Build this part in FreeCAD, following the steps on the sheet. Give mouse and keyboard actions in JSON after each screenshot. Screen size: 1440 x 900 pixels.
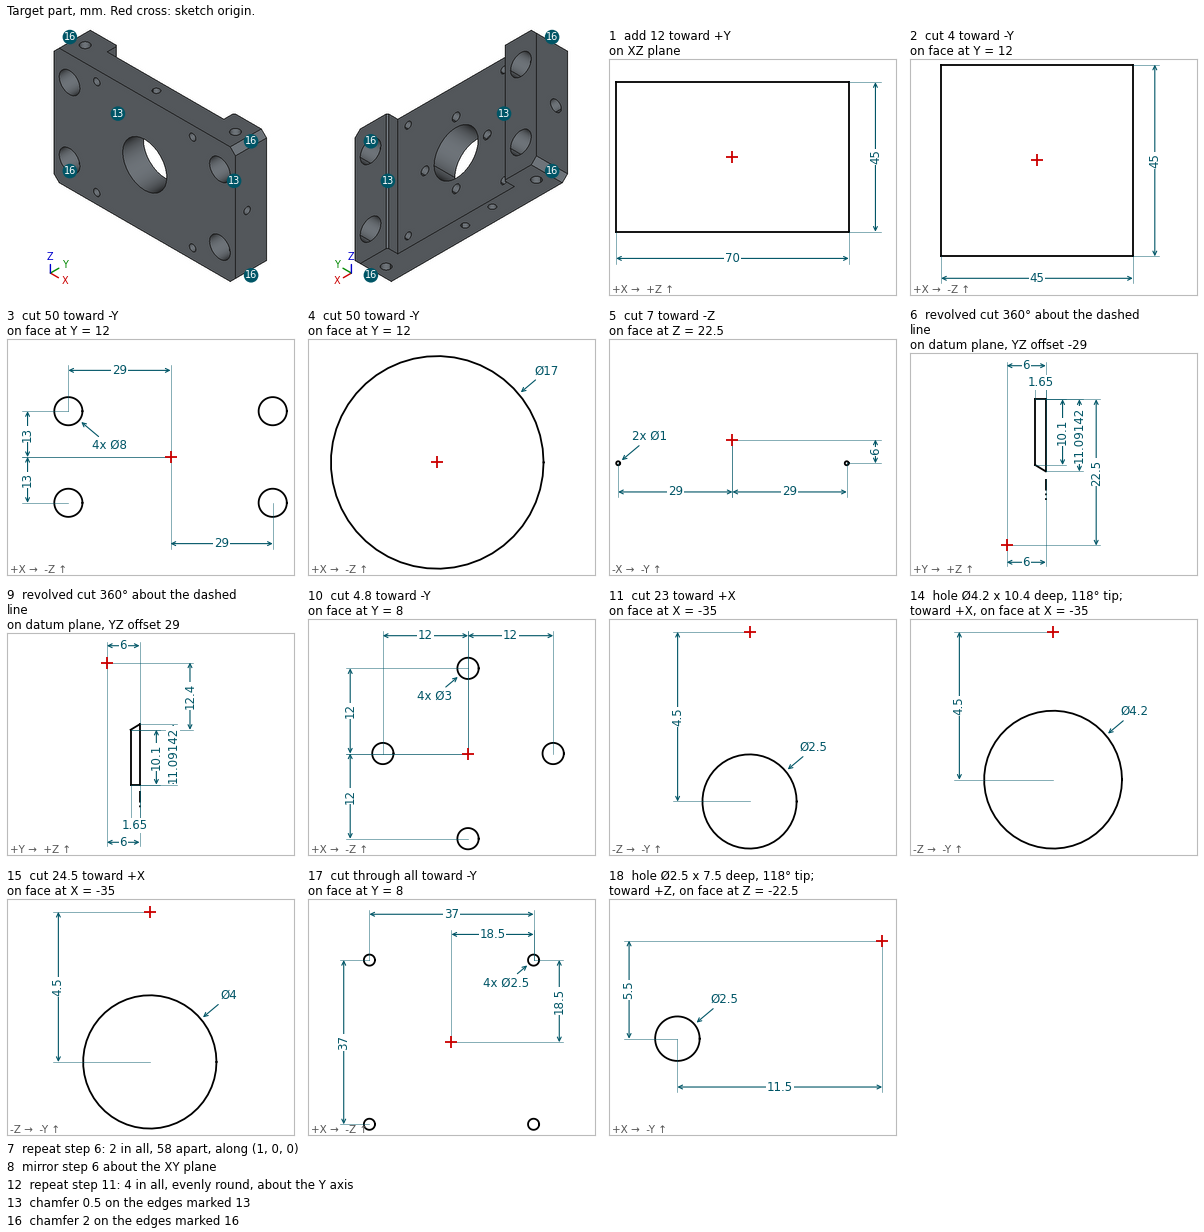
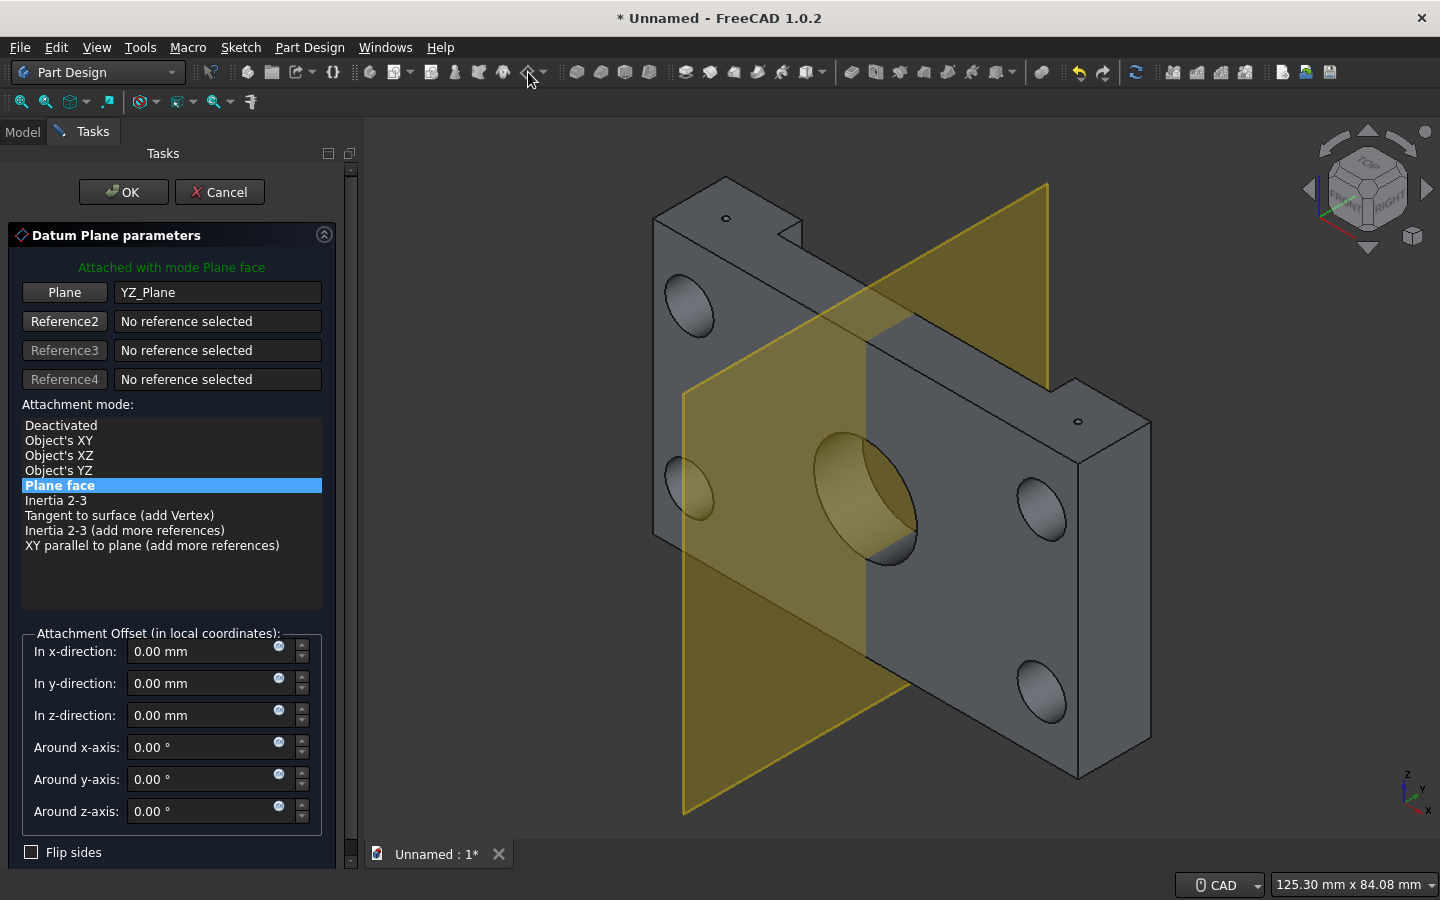
{"action": "triple_click", "coordinate": [210, 715]}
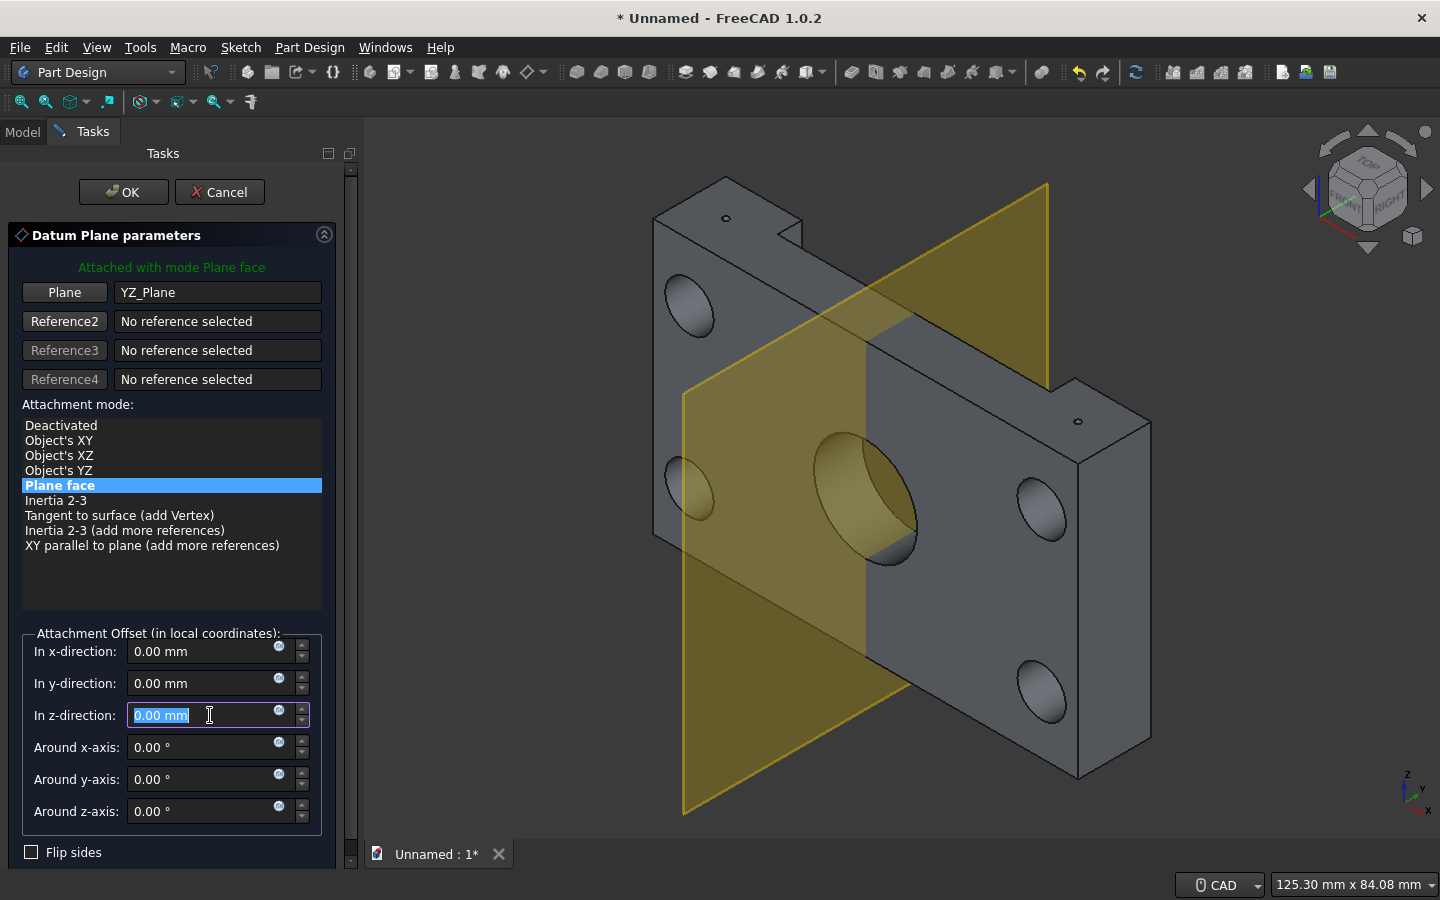
{"action": "type", "text": "-29"}
{"action": "key", "text": "Tab"}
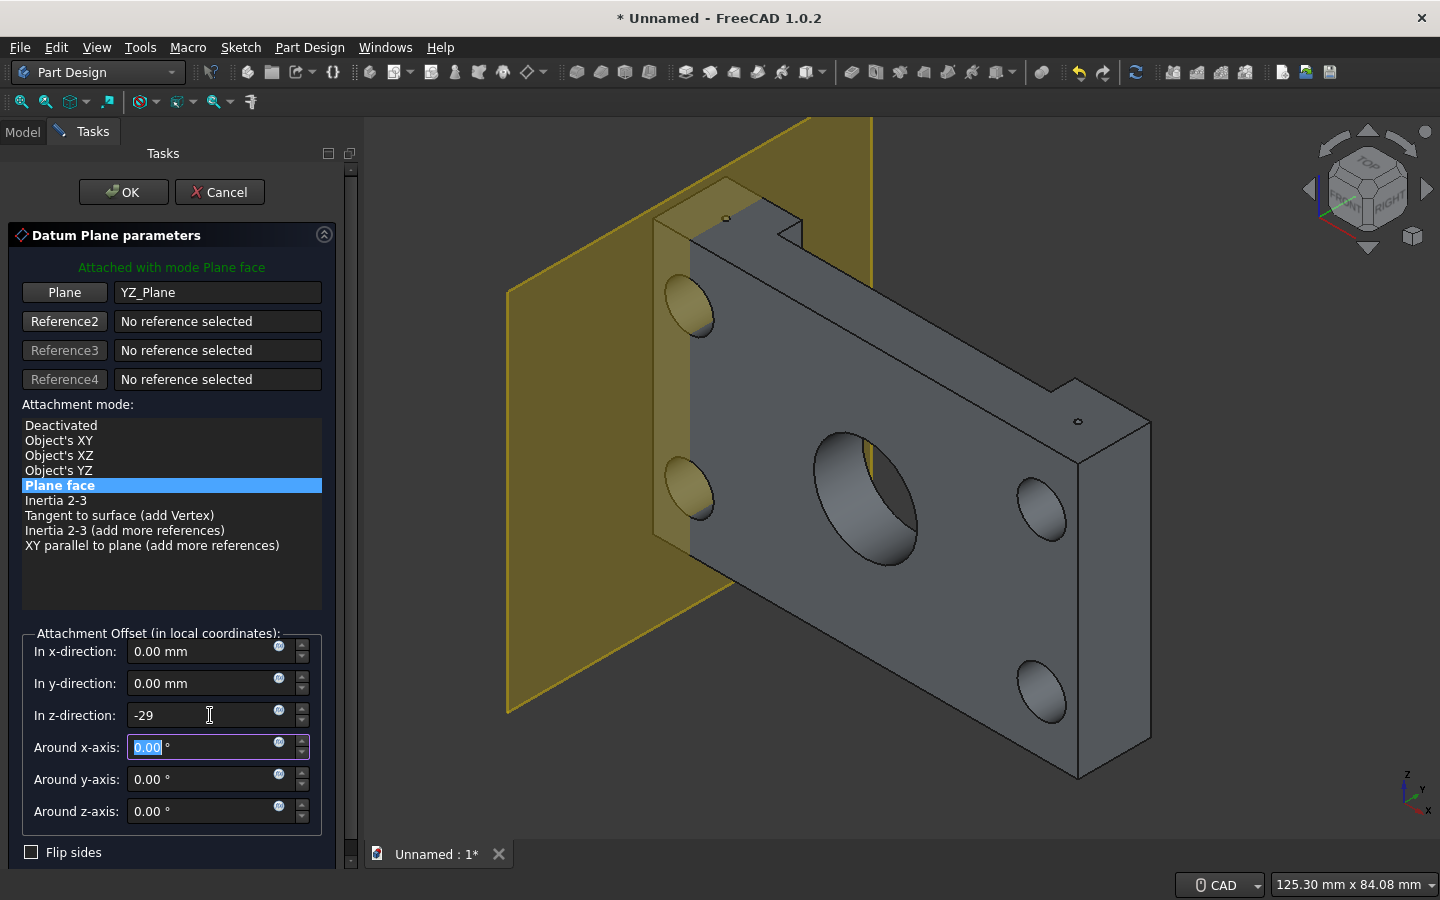
{"action": "left_click", "coordinate": [124, 192]}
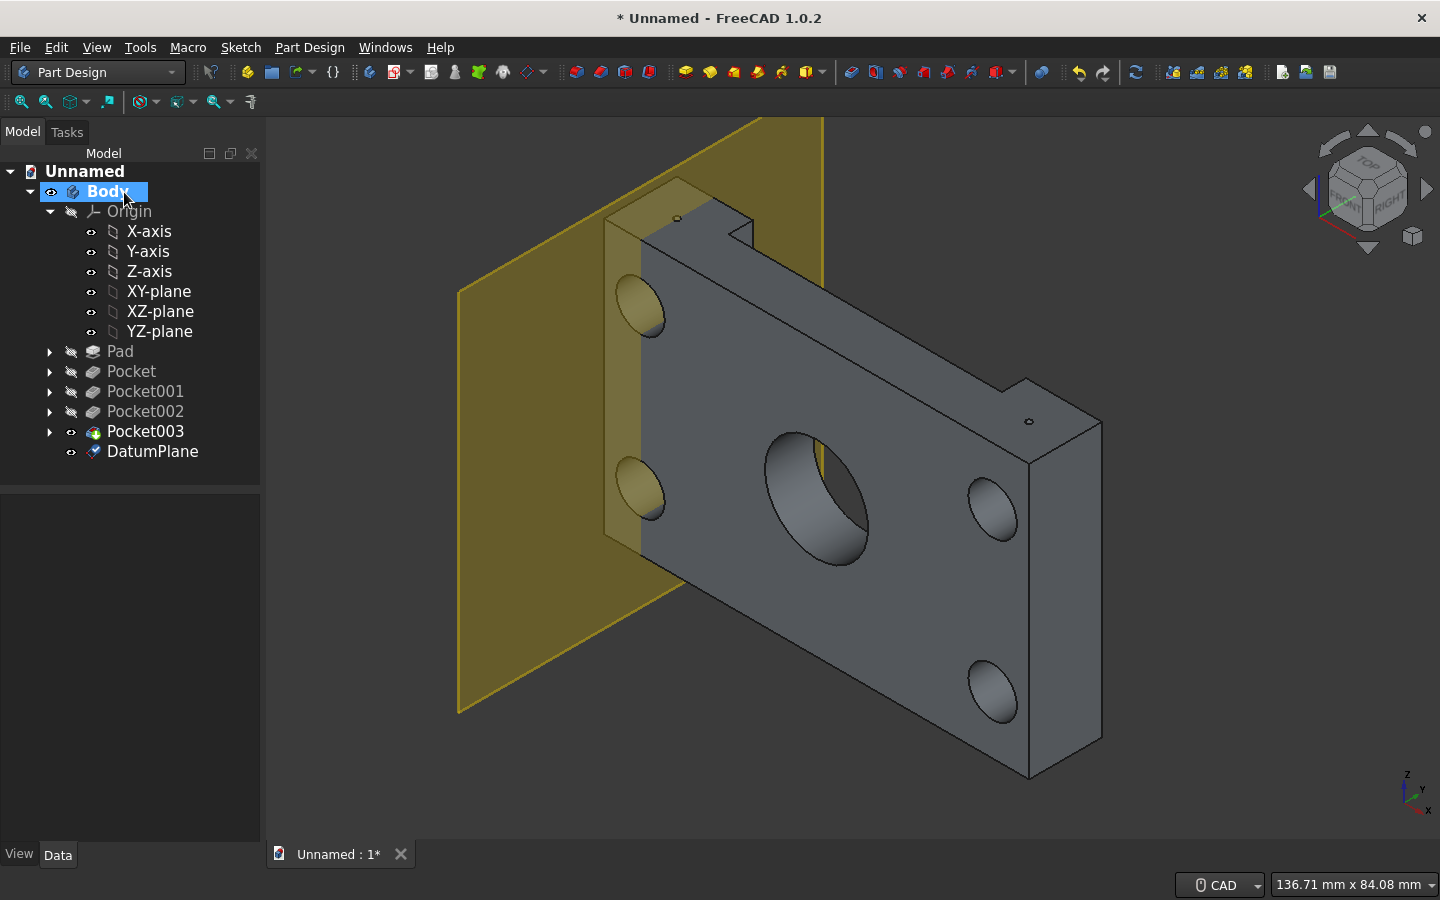
{"action": "left_click", "coordinate": [116, 452]}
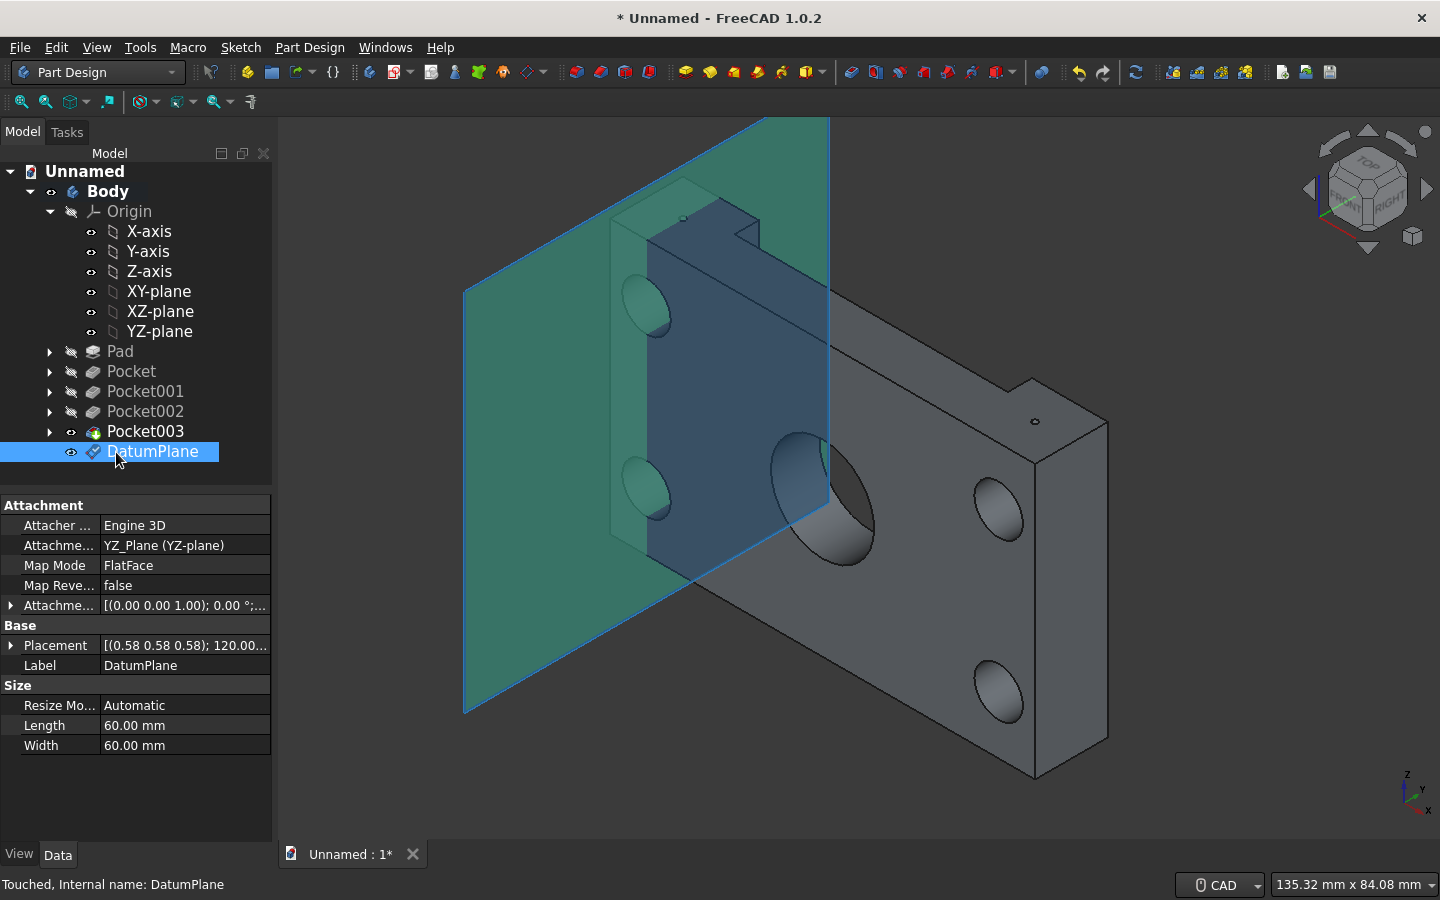
{"action": "left_click", "coordinate": [394, 72]}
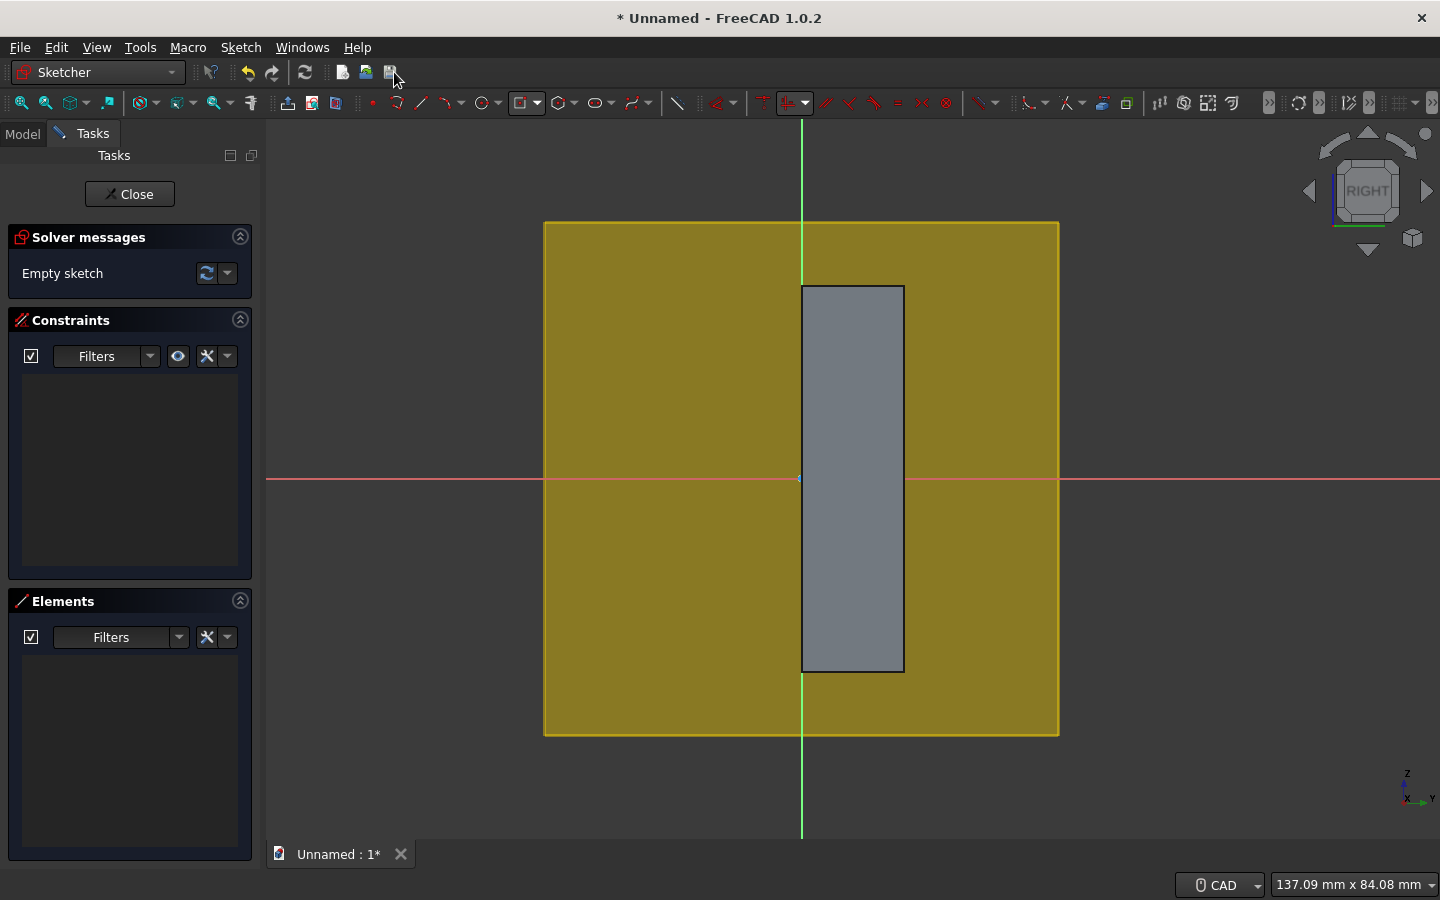
{"action": "left_click", "coordinate": [336, 104]}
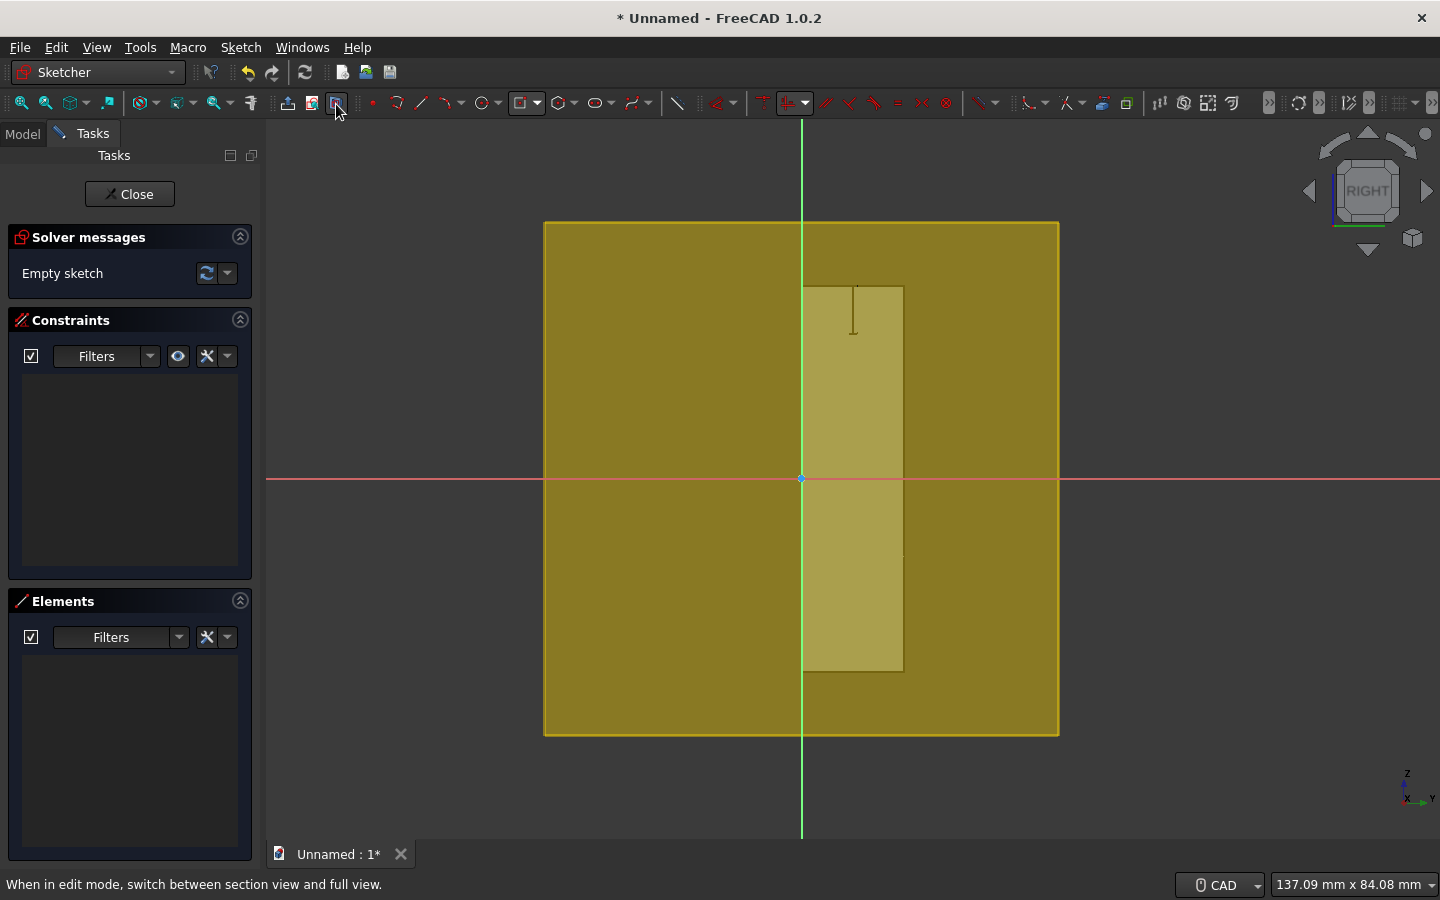
{"action": "scroll", "coordinate": [862, 304], "scroll_direction": "up", "scroll_amount": 4}